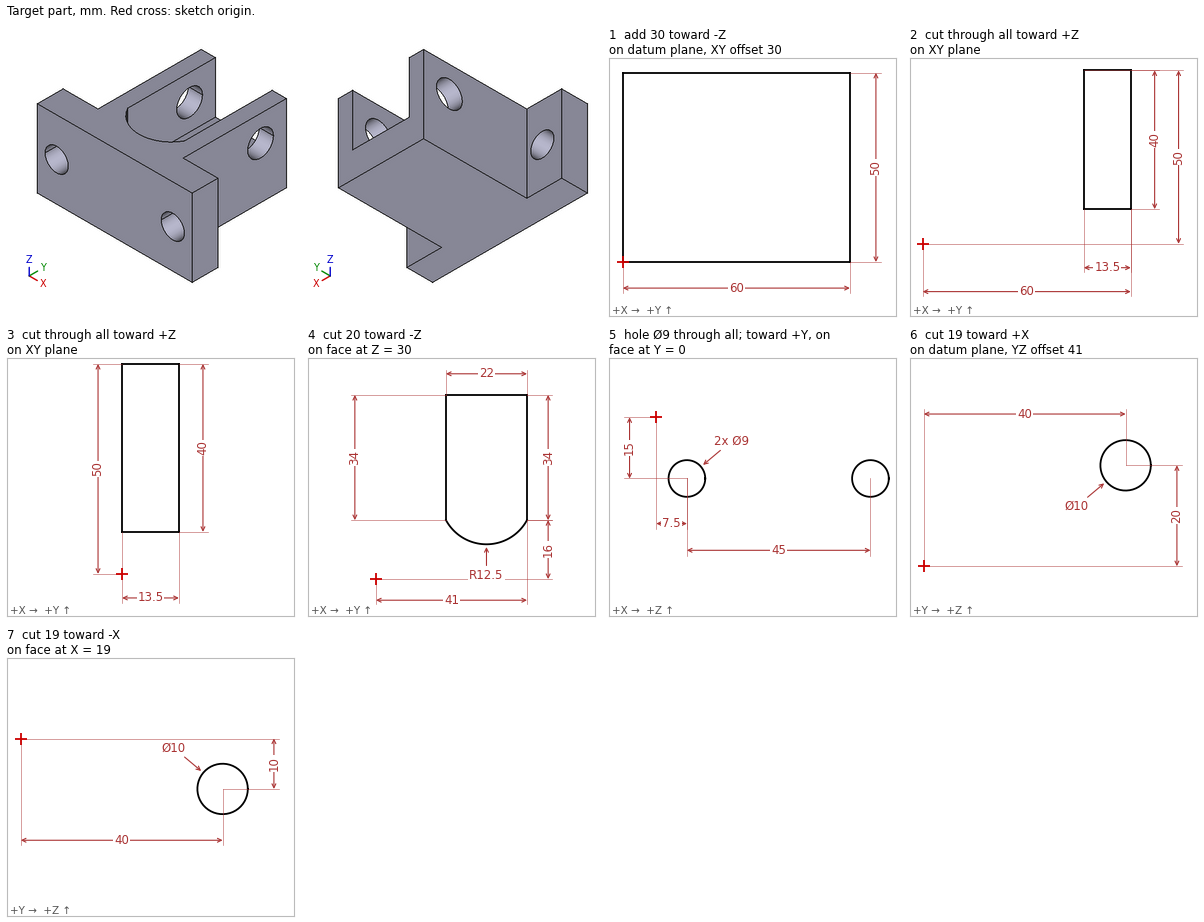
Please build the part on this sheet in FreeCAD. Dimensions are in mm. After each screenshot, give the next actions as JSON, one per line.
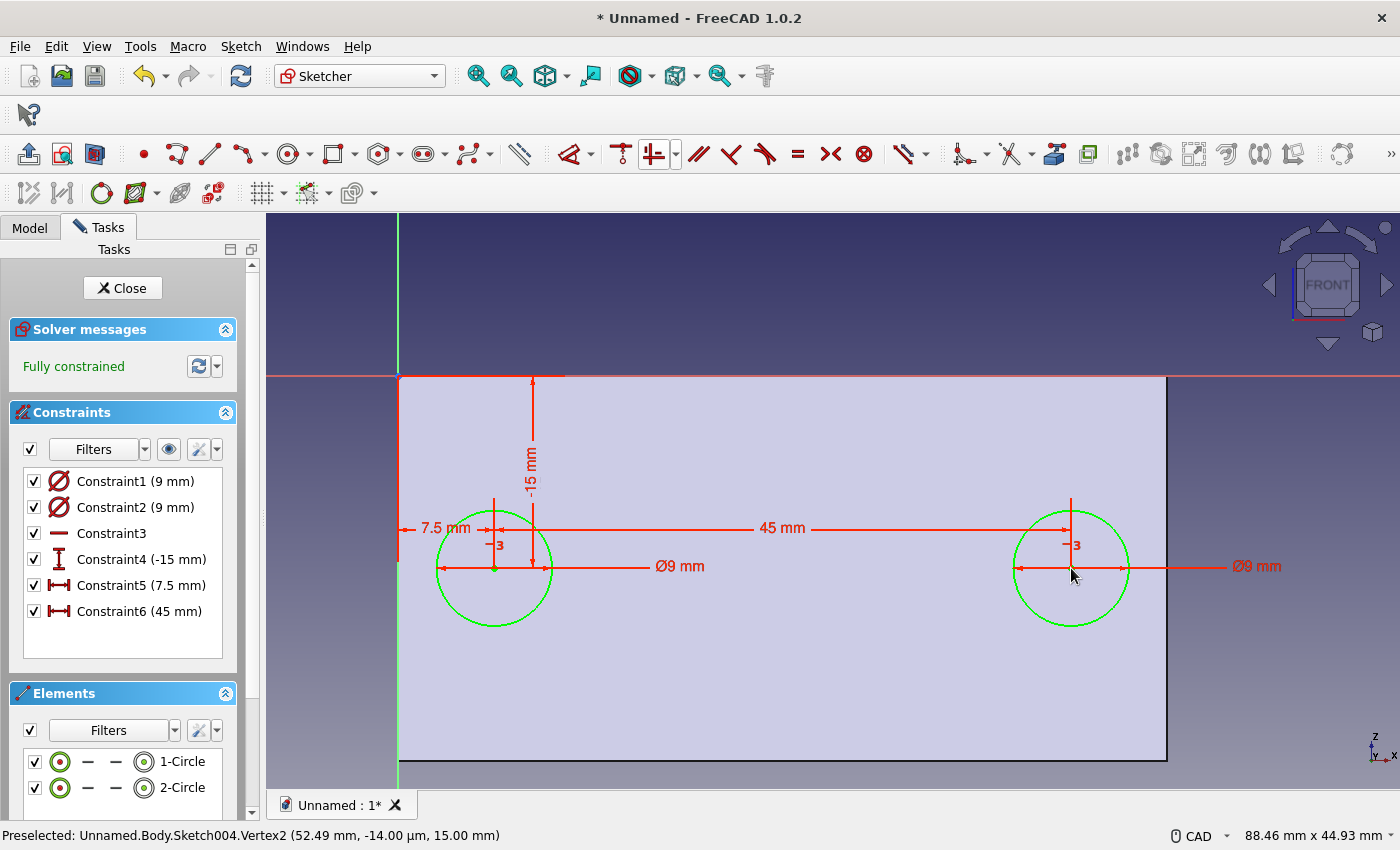
{"action": "left_click", "coordinate": [123, 288]}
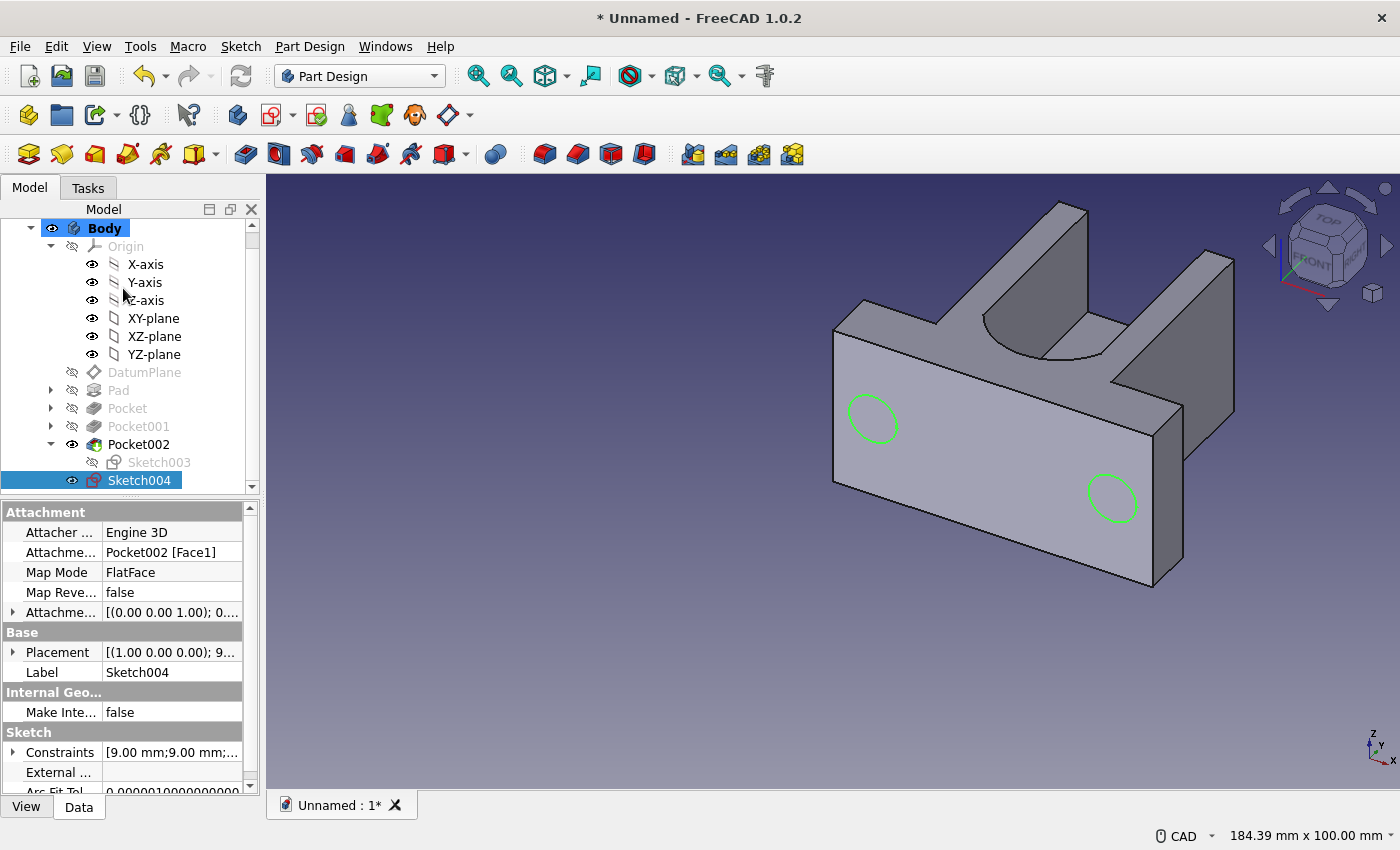
{"action": "left_click", "coordinate": [279, 154]}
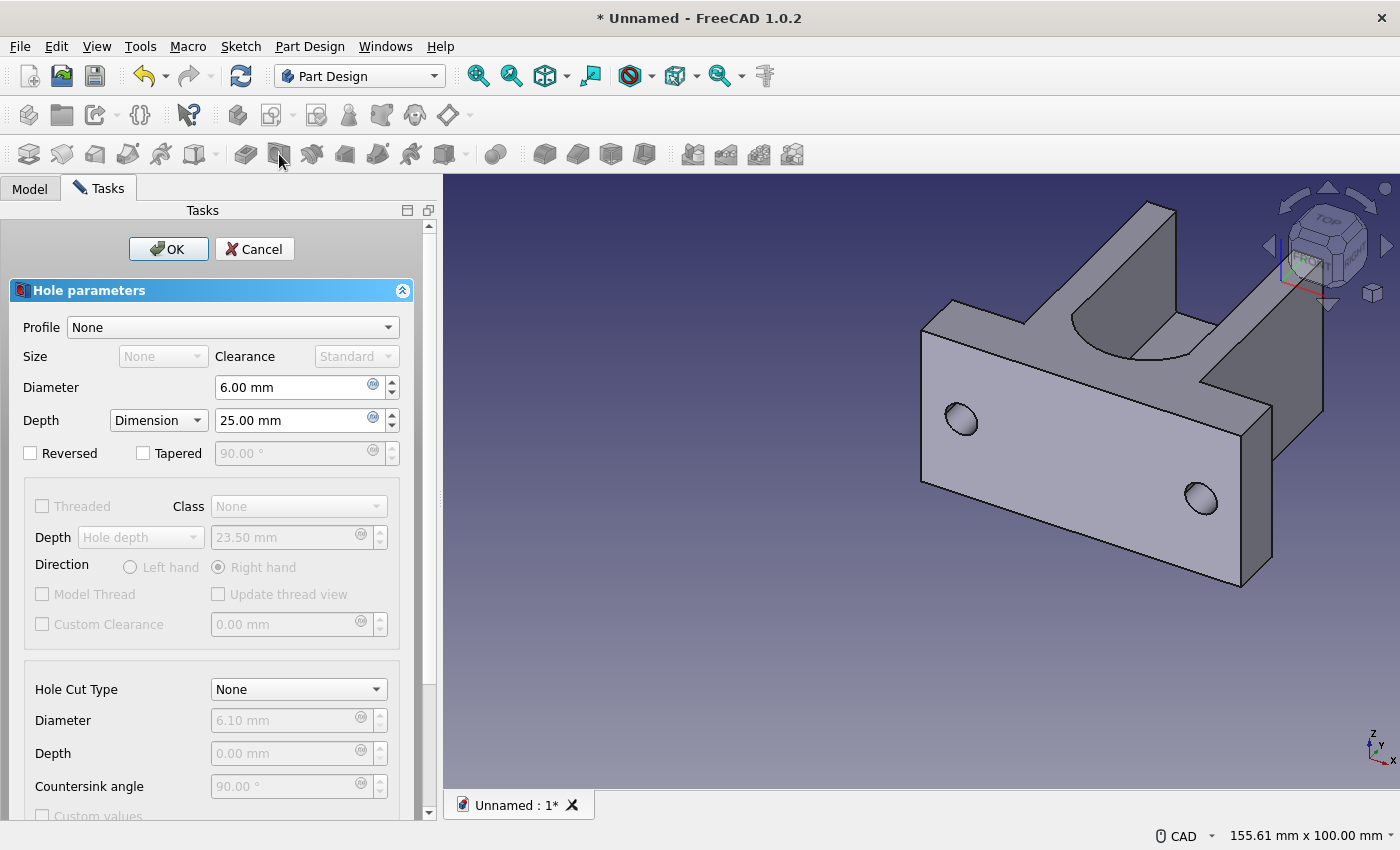
{"action": "triple_click", "coordinate": [300, 388]}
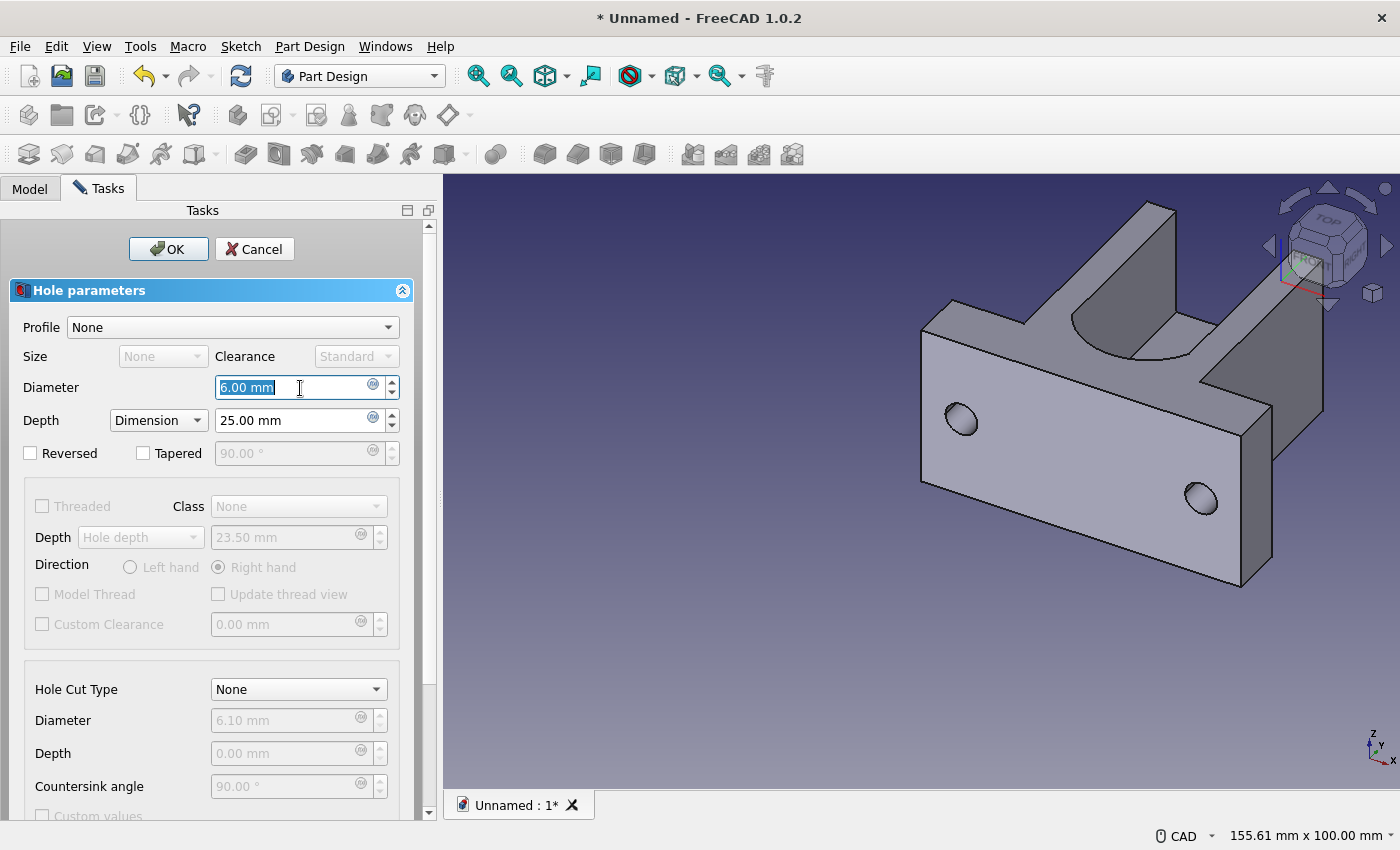
{"action": "type", "text": "9"}
{"action": "key", "text": "Tab"}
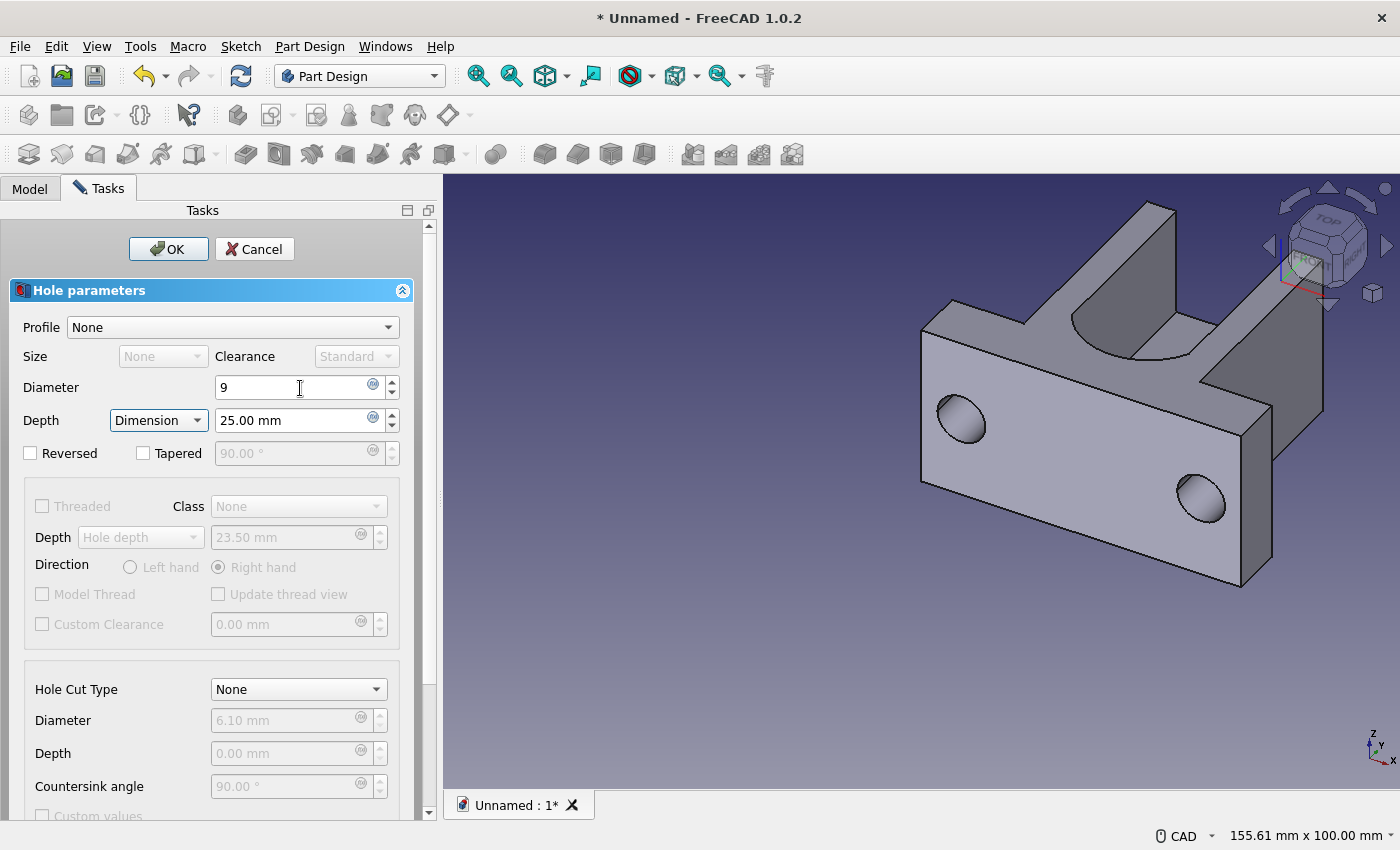
{"action": "left_click", "coordinate": [160, 420]}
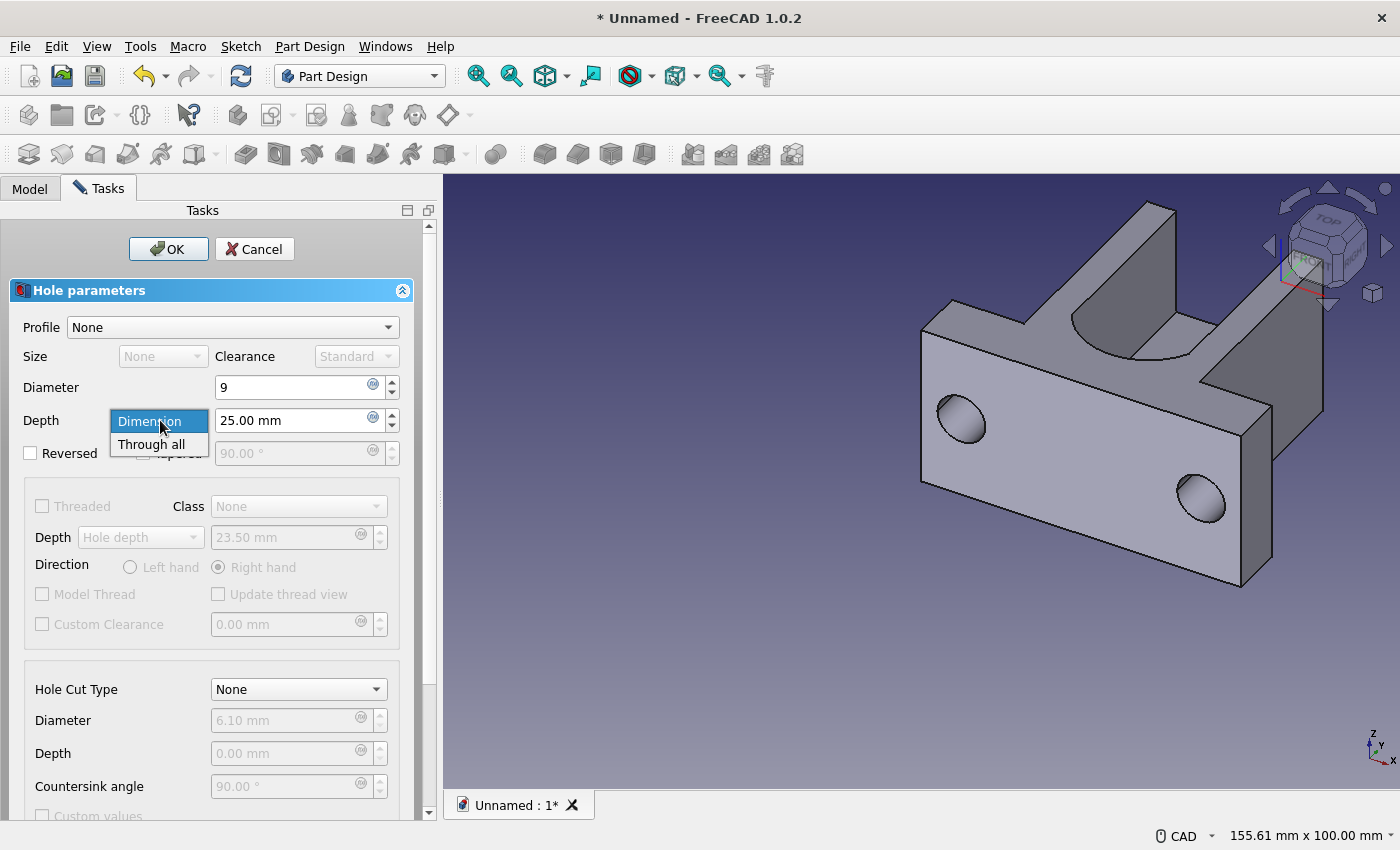
{"action": "left_click", "coordinate": [158, 444]}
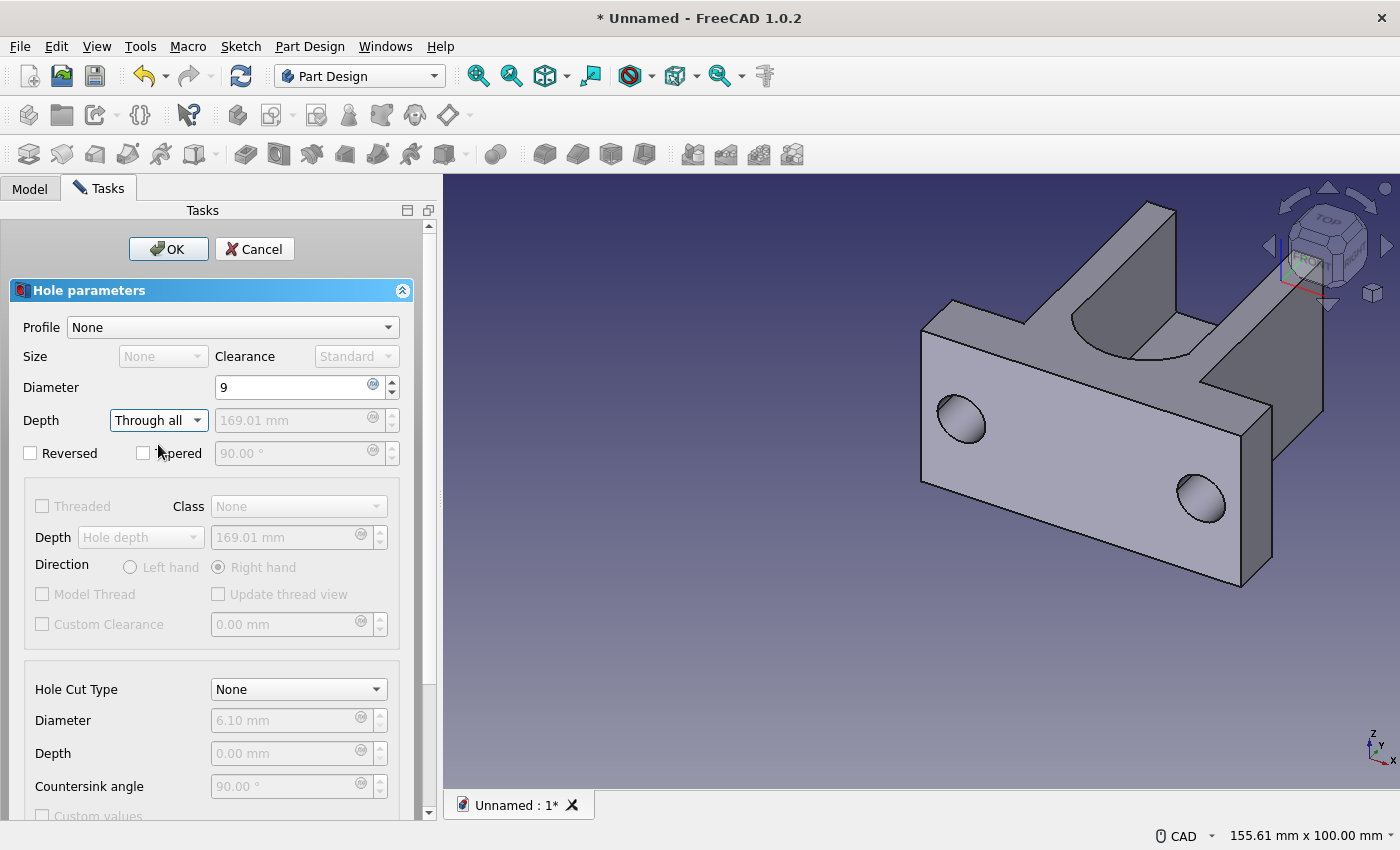
{"action": "left_click", "coordinate": [169, 249]}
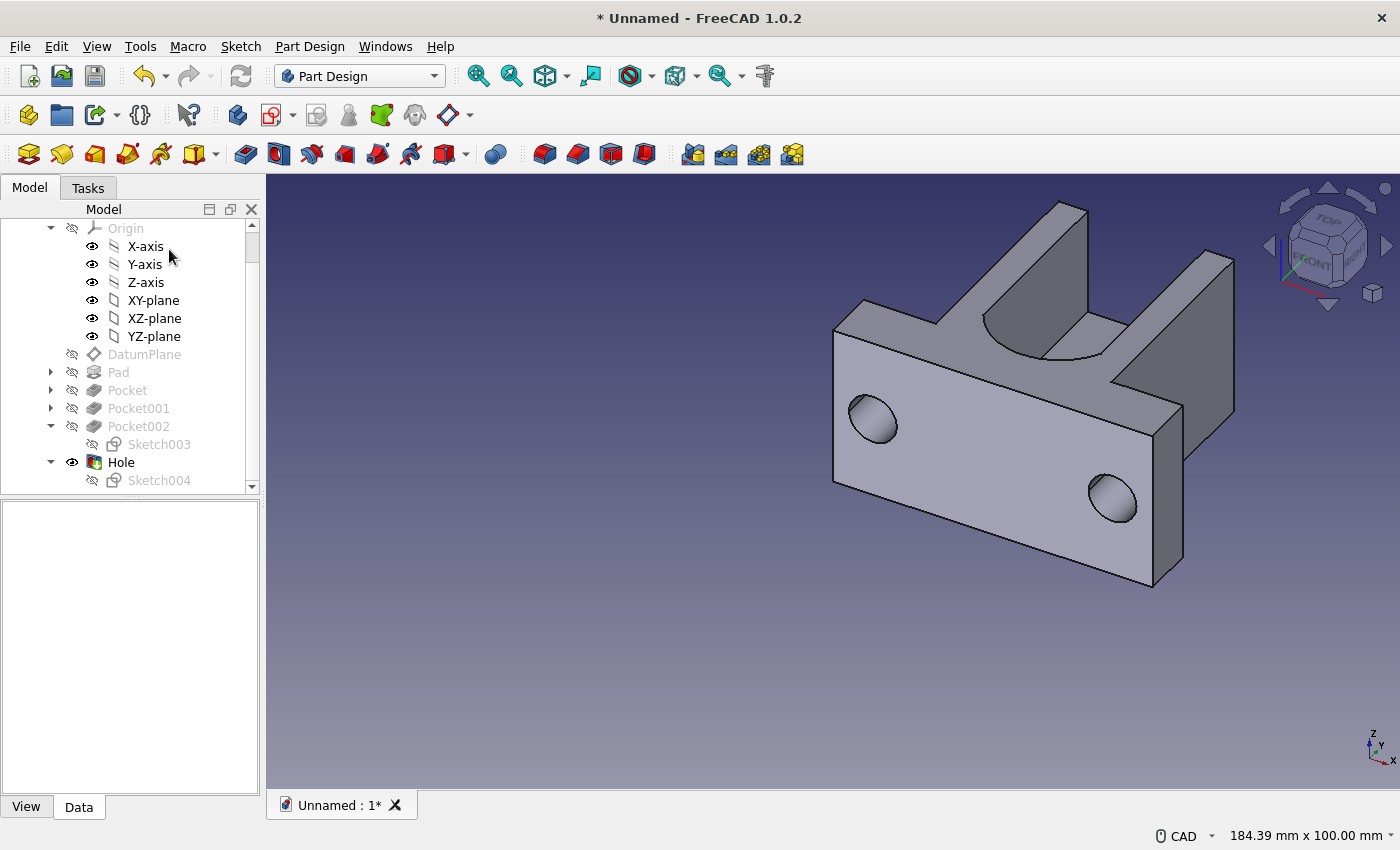
{"action": "left_click", "coordinate": [137, 336]}